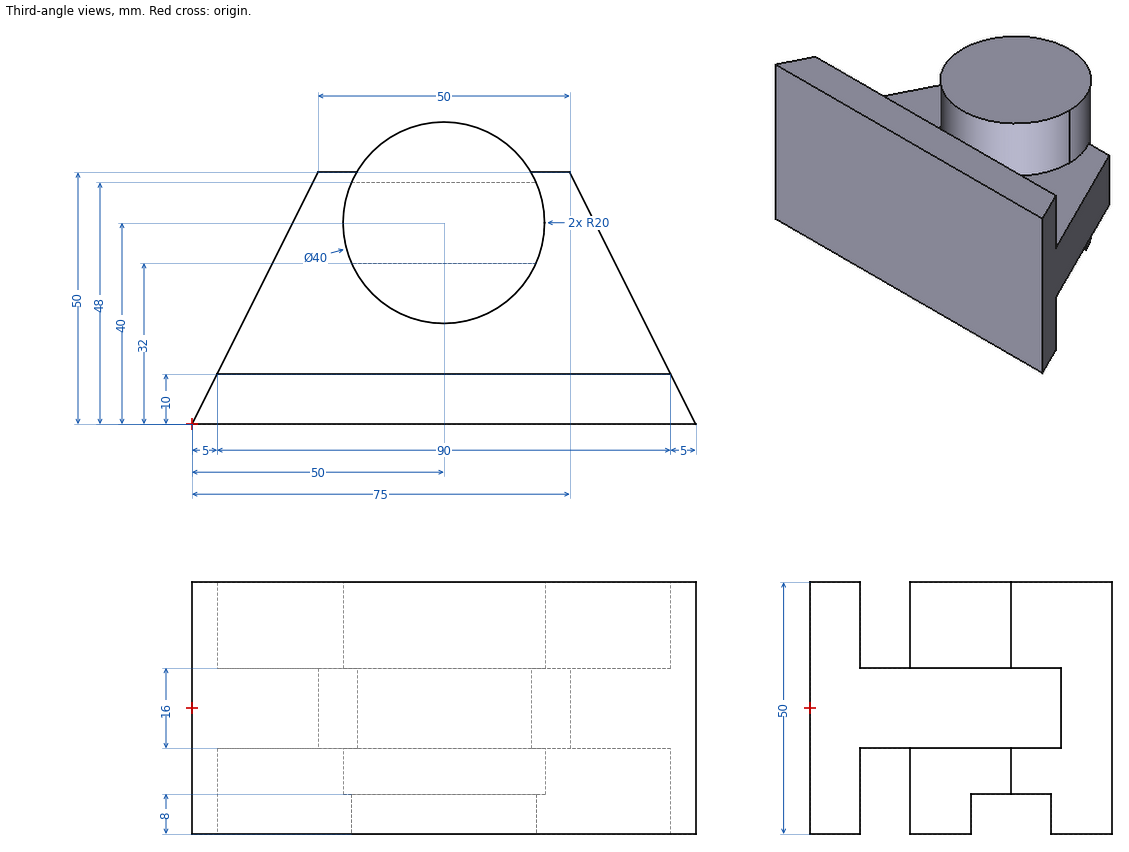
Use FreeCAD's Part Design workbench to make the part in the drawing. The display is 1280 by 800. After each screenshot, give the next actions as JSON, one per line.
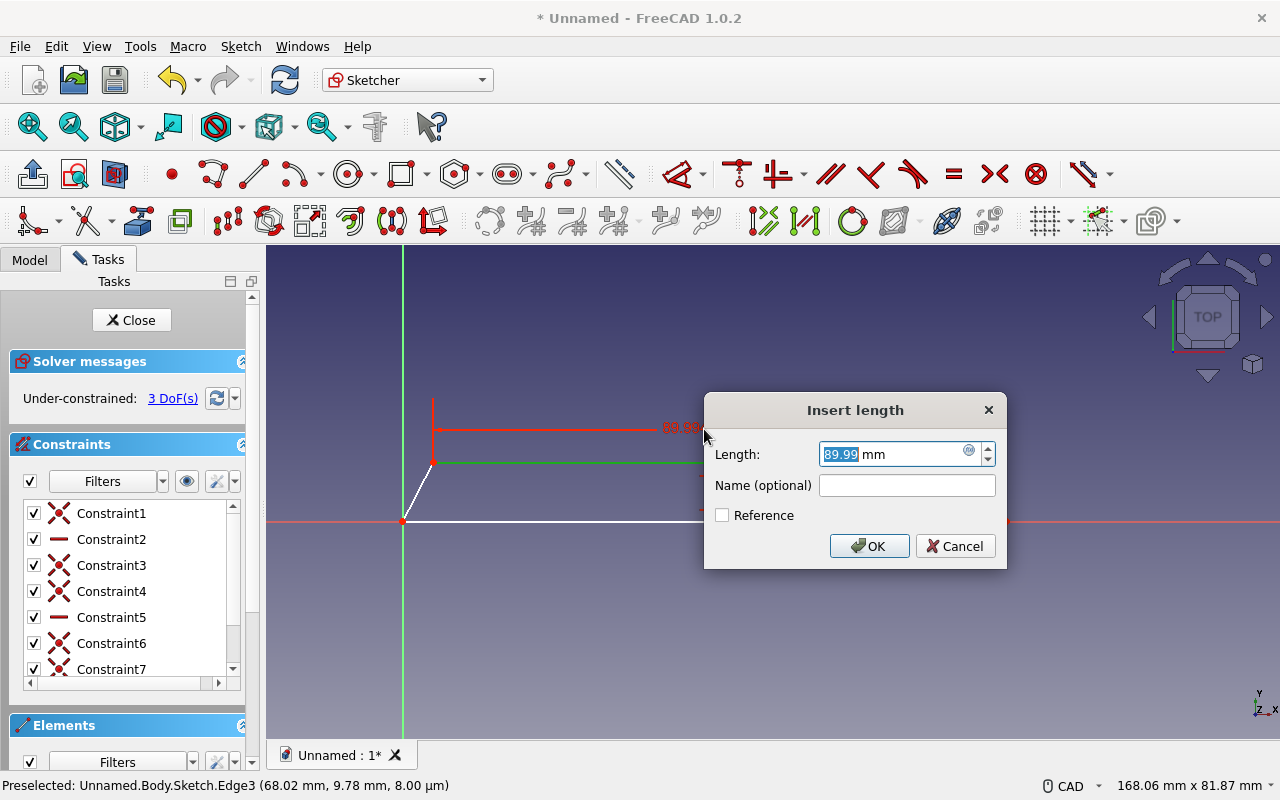
{"action": "type", "text": "90"}
{"action": "key", "text": "Return"}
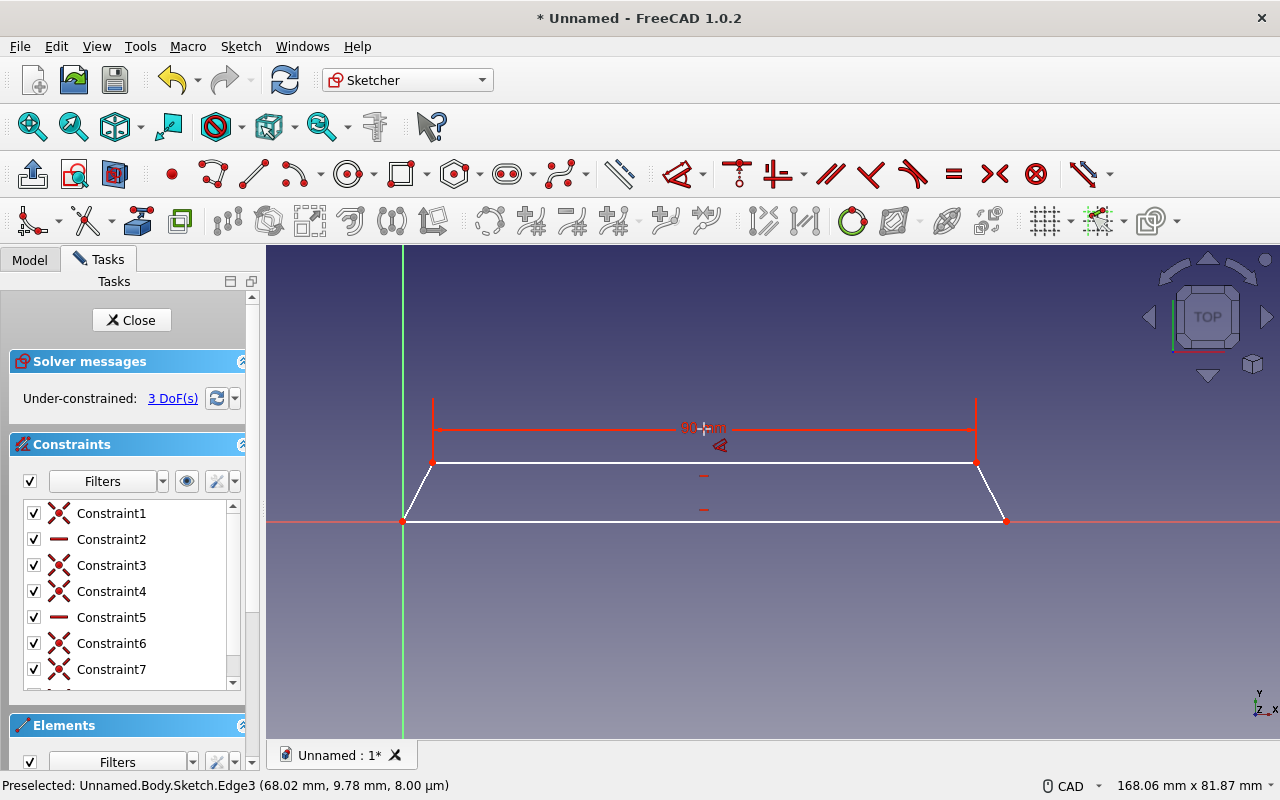
{"action": "scroll", "coordinate": [433, 463], "scroll_direction": "up", "scroll_amount": 2}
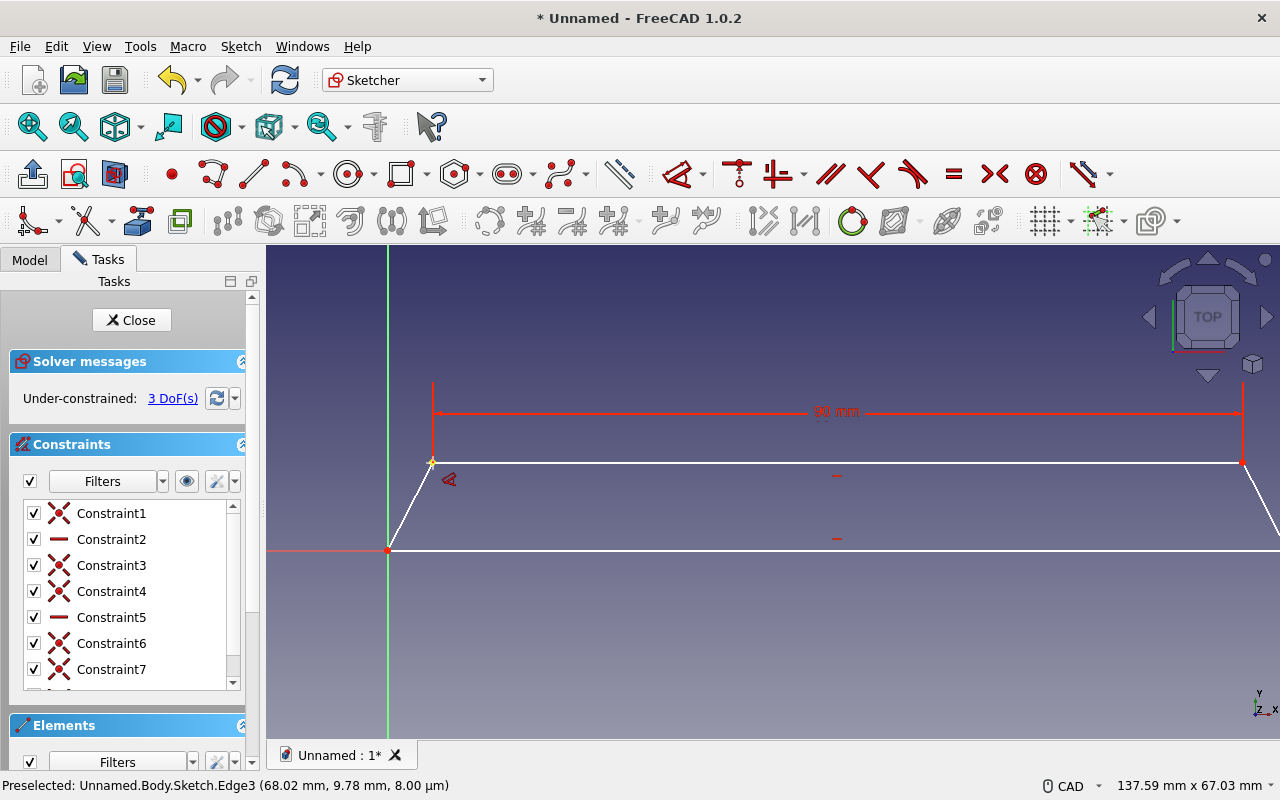
{"action": "left_click", "coordinate": [433, 463]}
{"action": "left_click", "coordinate": [410, 585]}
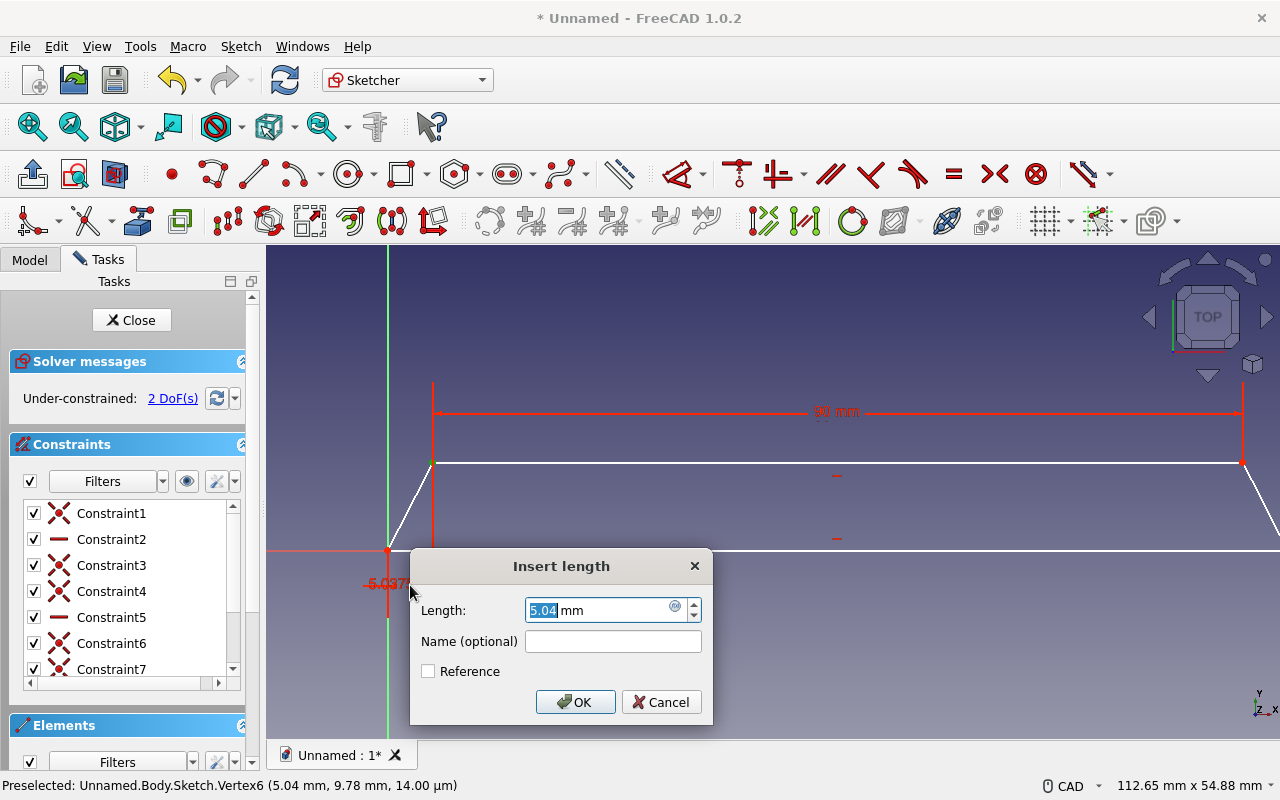
{"action": "type", "text": "5"}
{"action": "key", "text": "Return"}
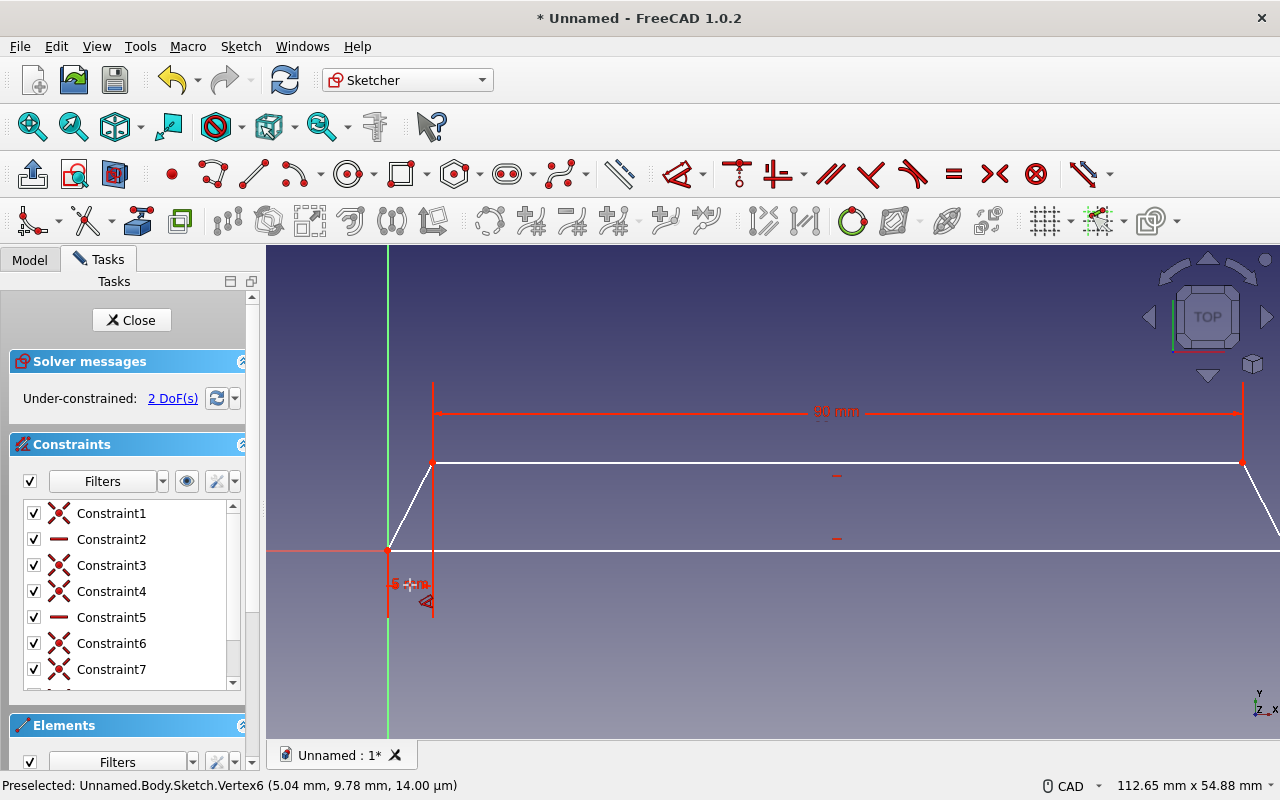
{"action": "scroll", "coordinate": [434, 464], "scroll_direction": "down", "scroll_amount": 2}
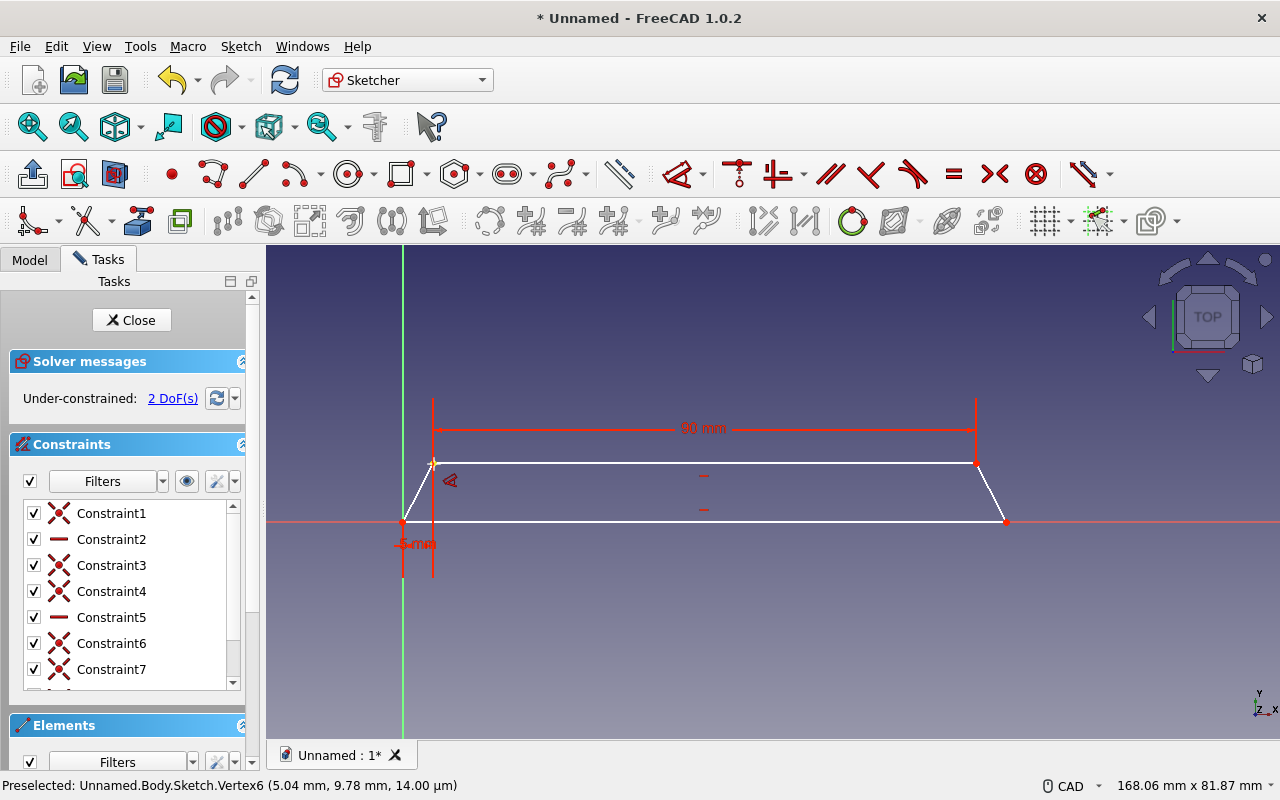
{"action": "scroll", "coordinate": [997, 505], "scroll_direction": "up", "scroll_amount": 2}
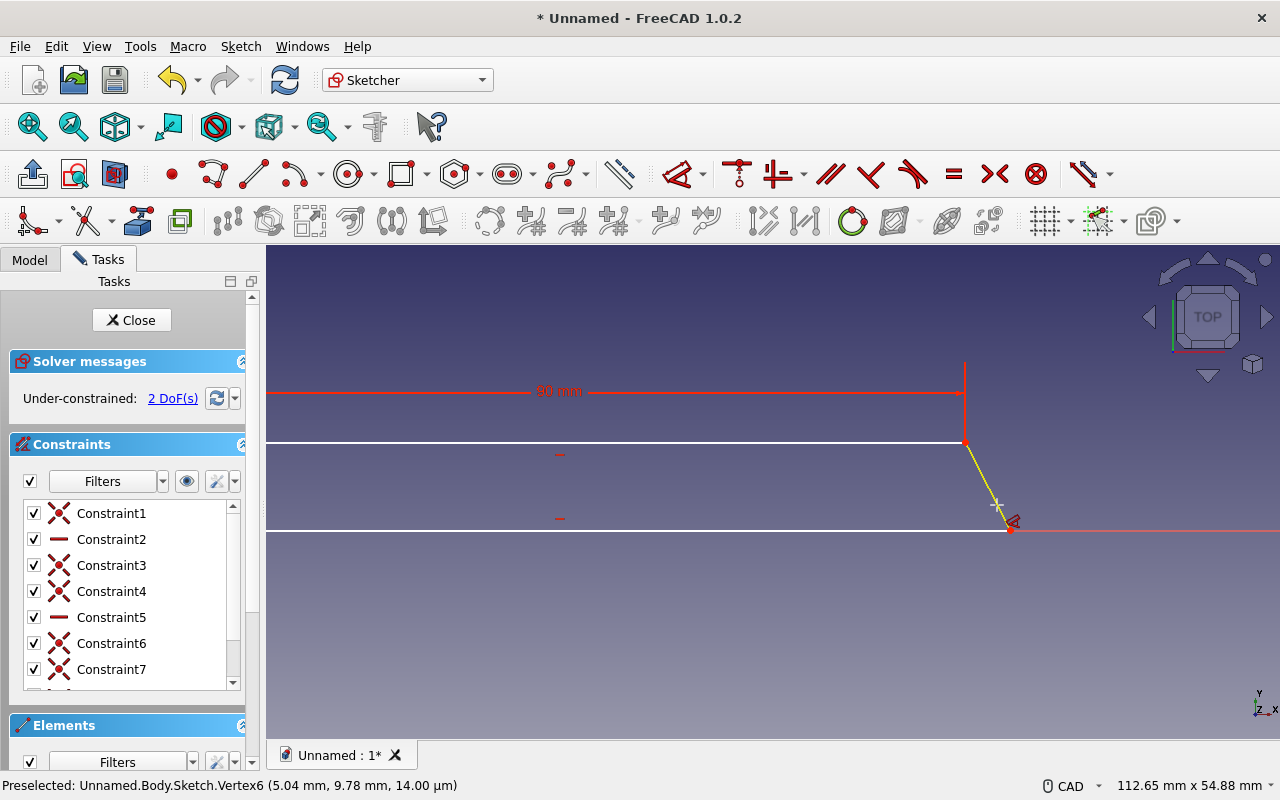
{"action": "left_click", "coordinate": [997, 504]}
{"action": "left_click", "coordinate": [988, 565]}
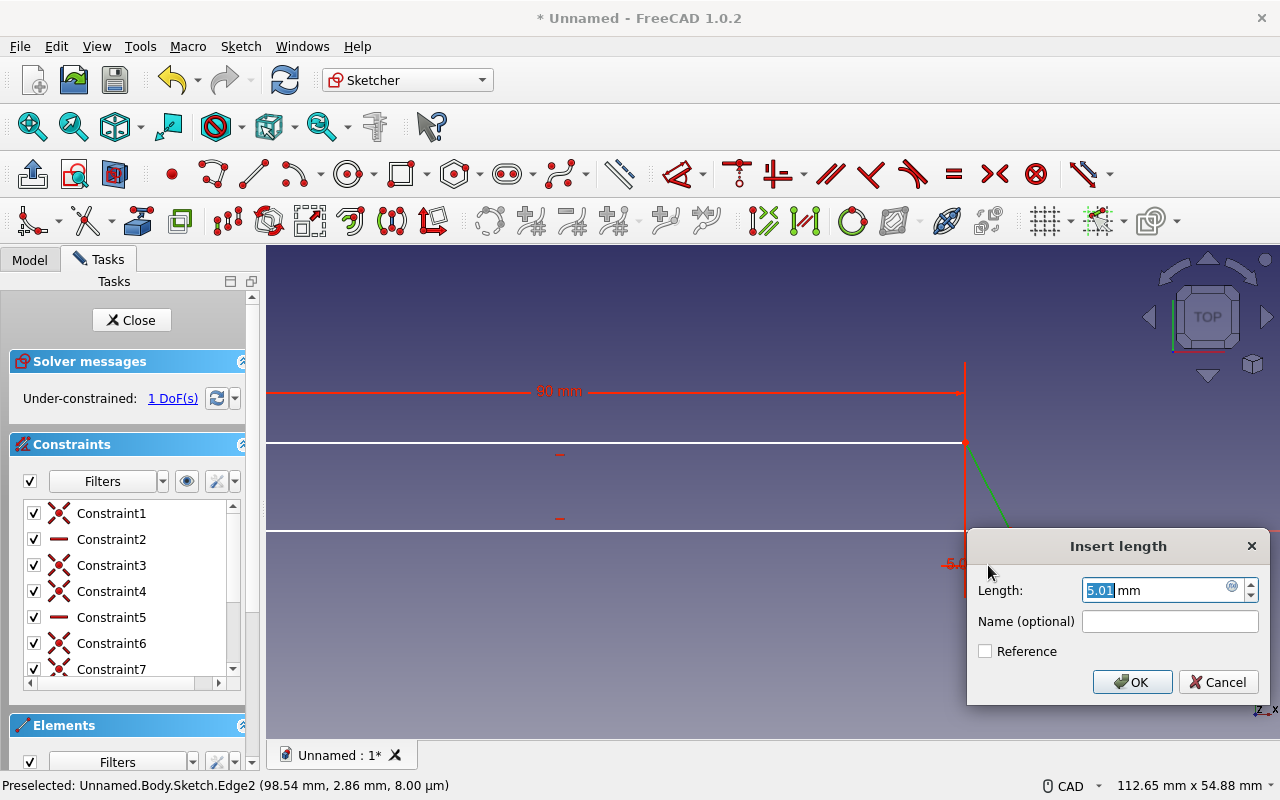
{"action": "type", "text": "5"}
{"action": "key", "text": "Return"}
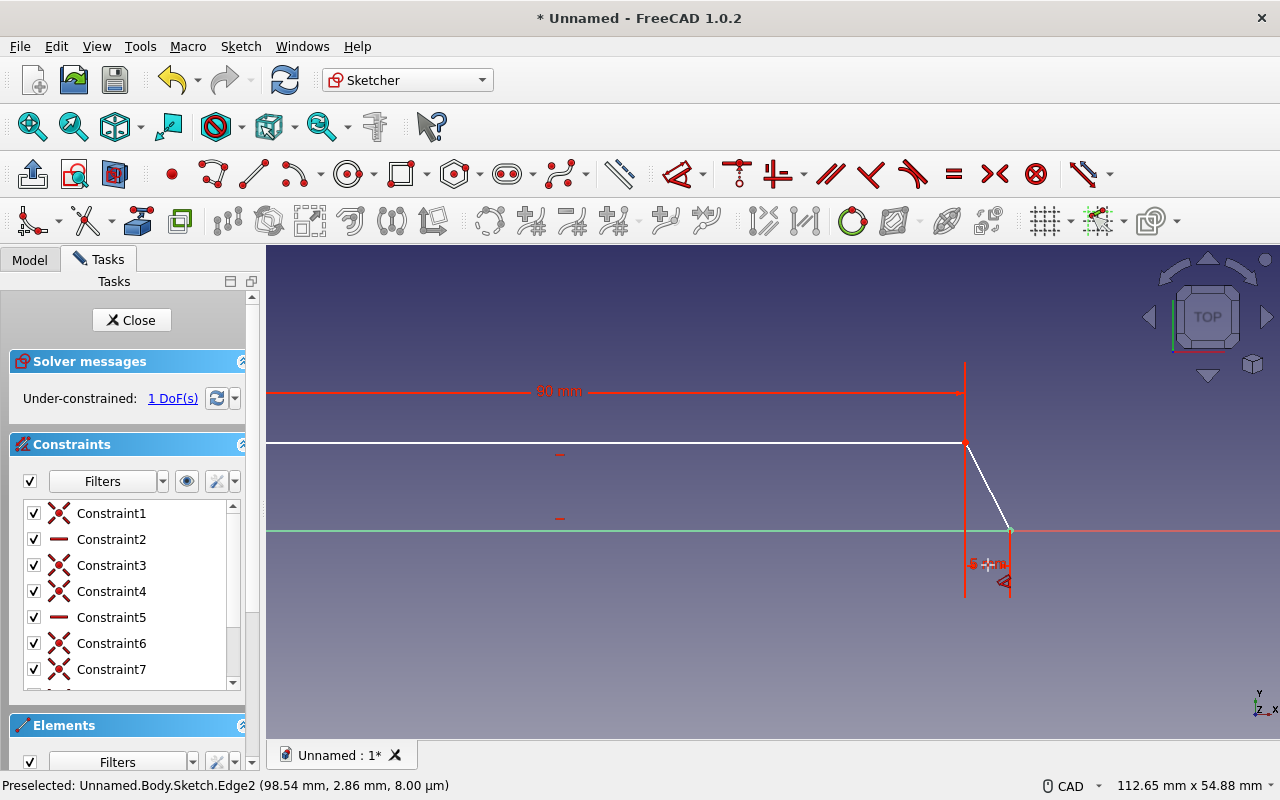
{"action": "left_click", "coordinate": [965, 443]}
{"action": "left_click", "coordinate": [999, 466]}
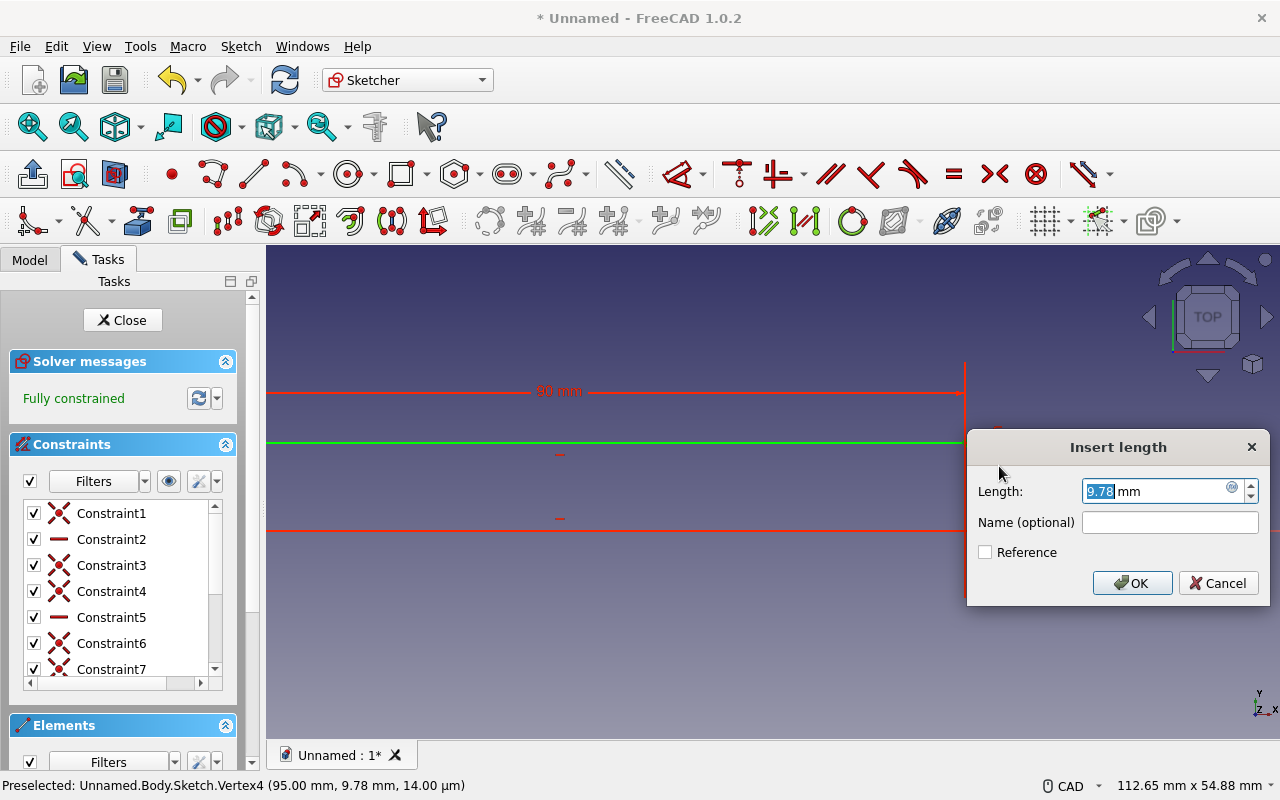
{"action": "type", "text": "10"}
{"action": "key", "text": "Return"}
{"action": "key", "text": "Escape"}